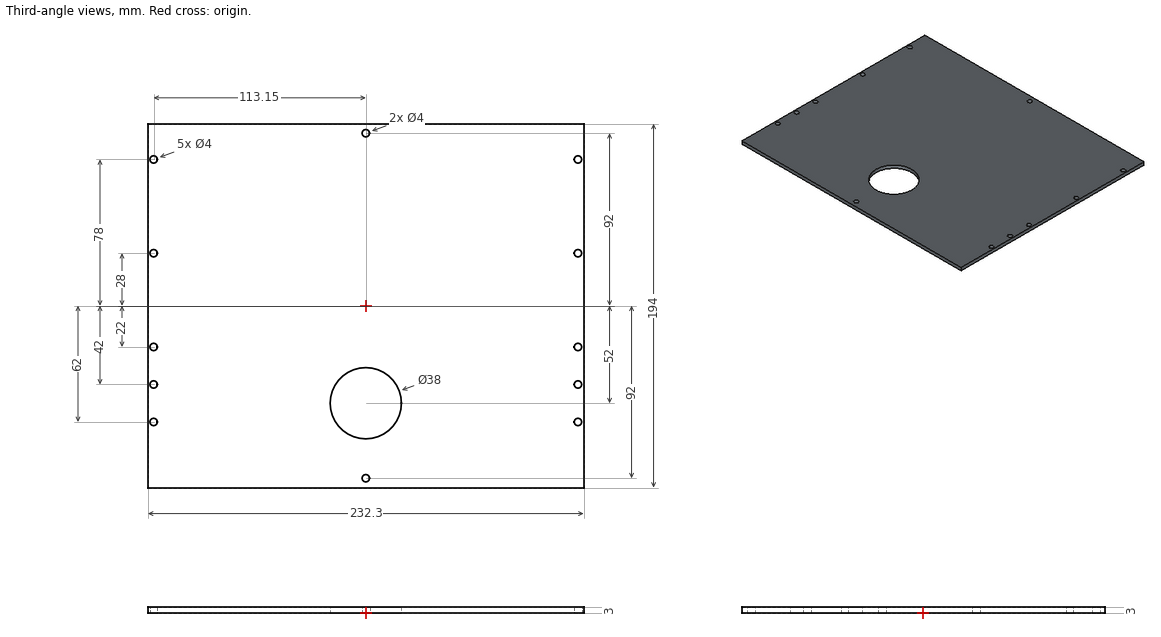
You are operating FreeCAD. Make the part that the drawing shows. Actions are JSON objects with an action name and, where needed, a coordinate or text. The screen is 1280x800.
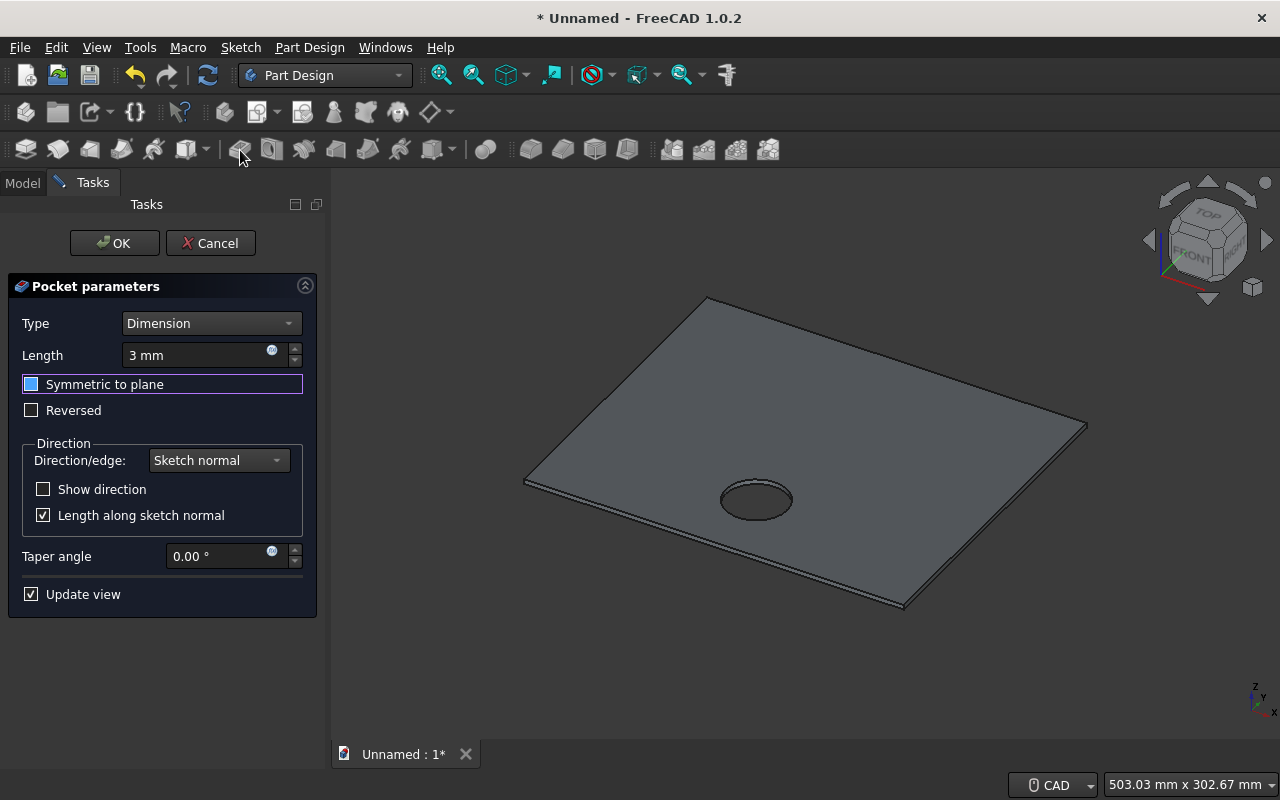
{"action": "left_click", "coordinate": [115, 243]}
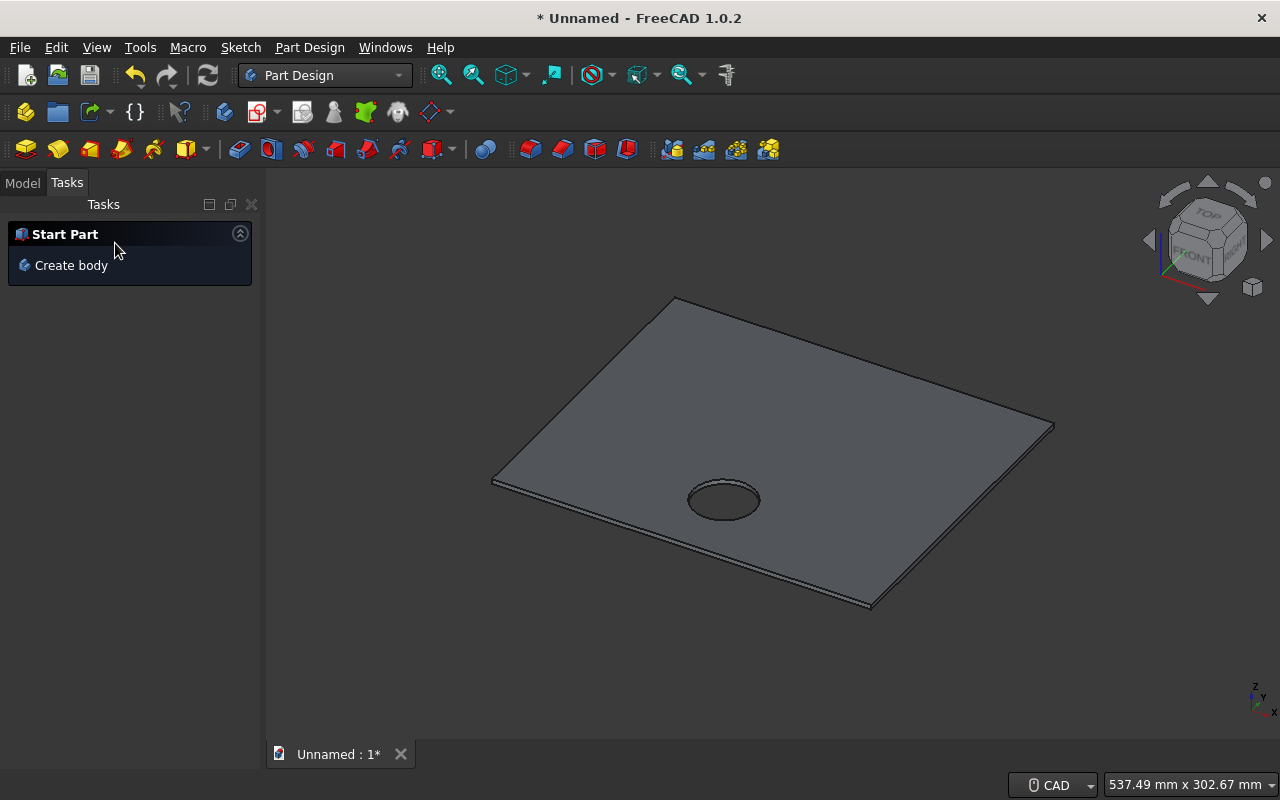
{"action": "left_click", "coordinate": [853, 442]}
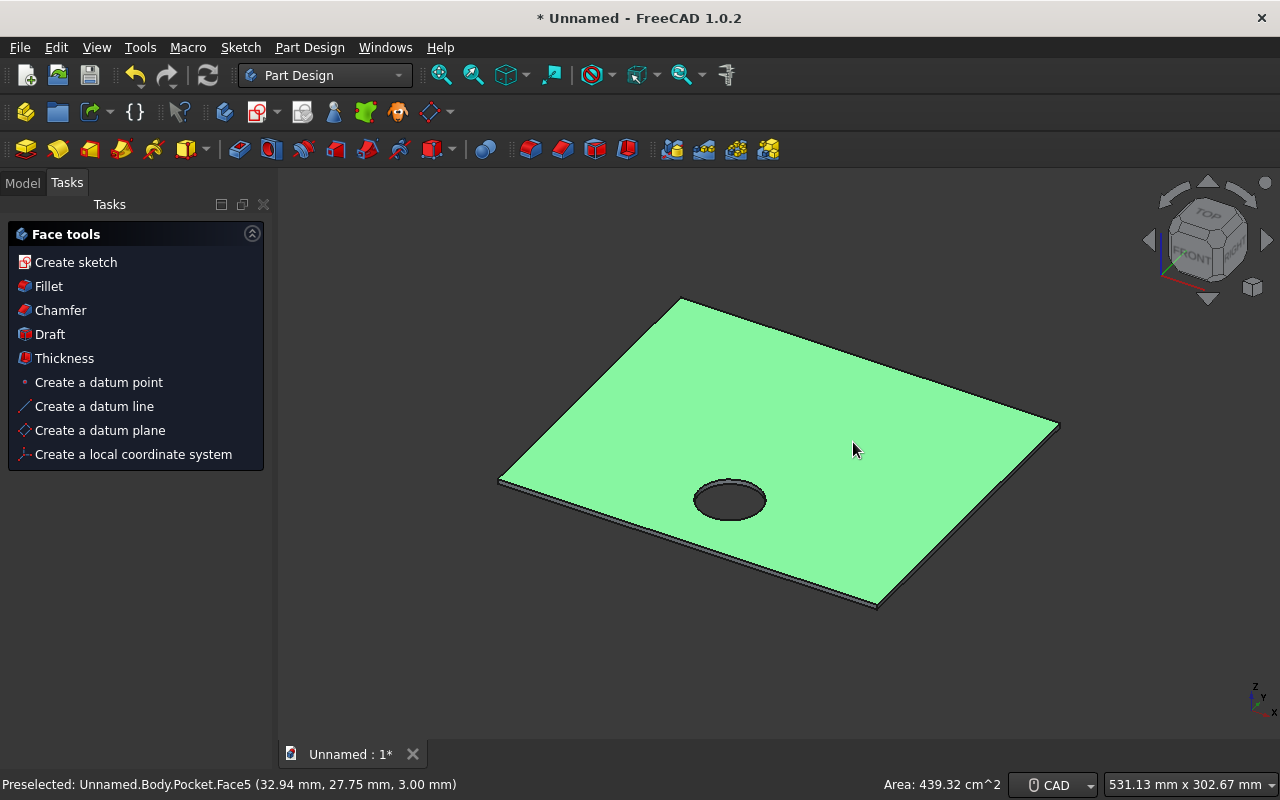
{"action": "left_click", "coordinate": [258, 112]}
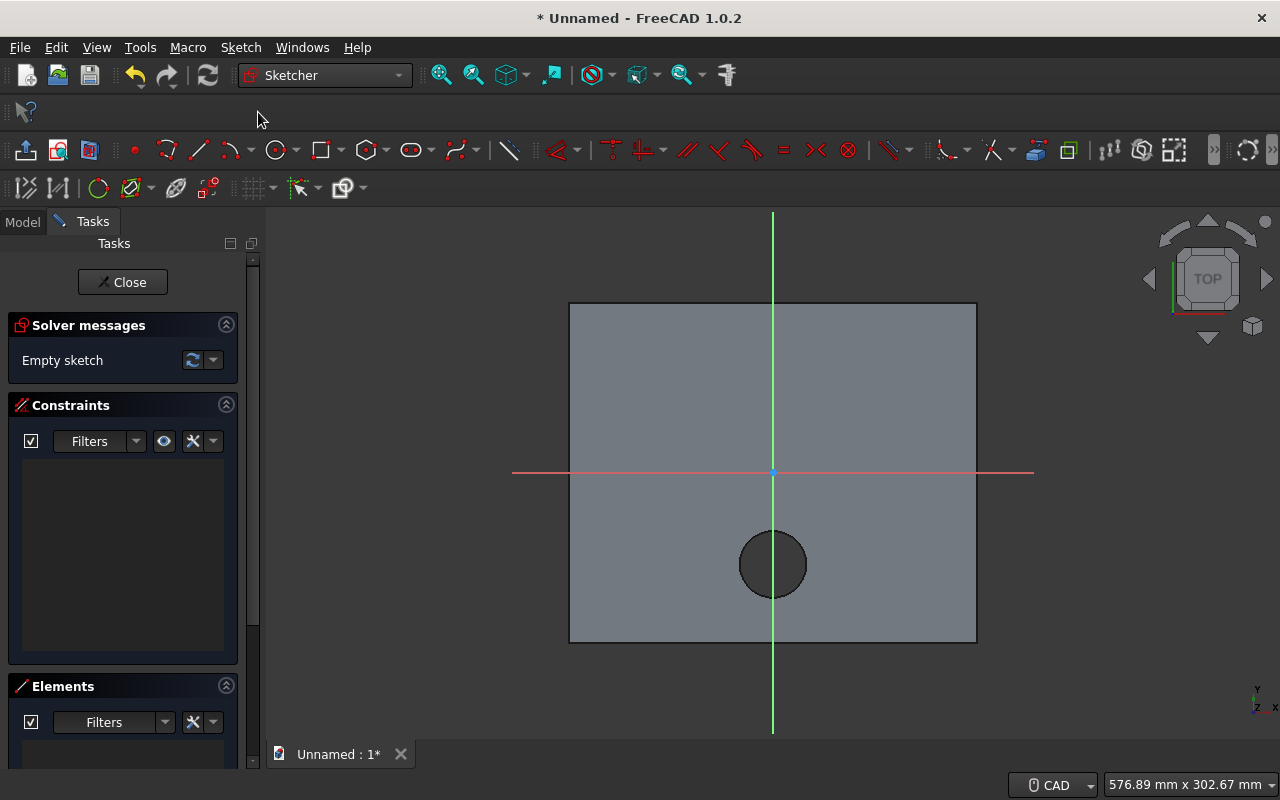
{"action": "key", "text": "g c"}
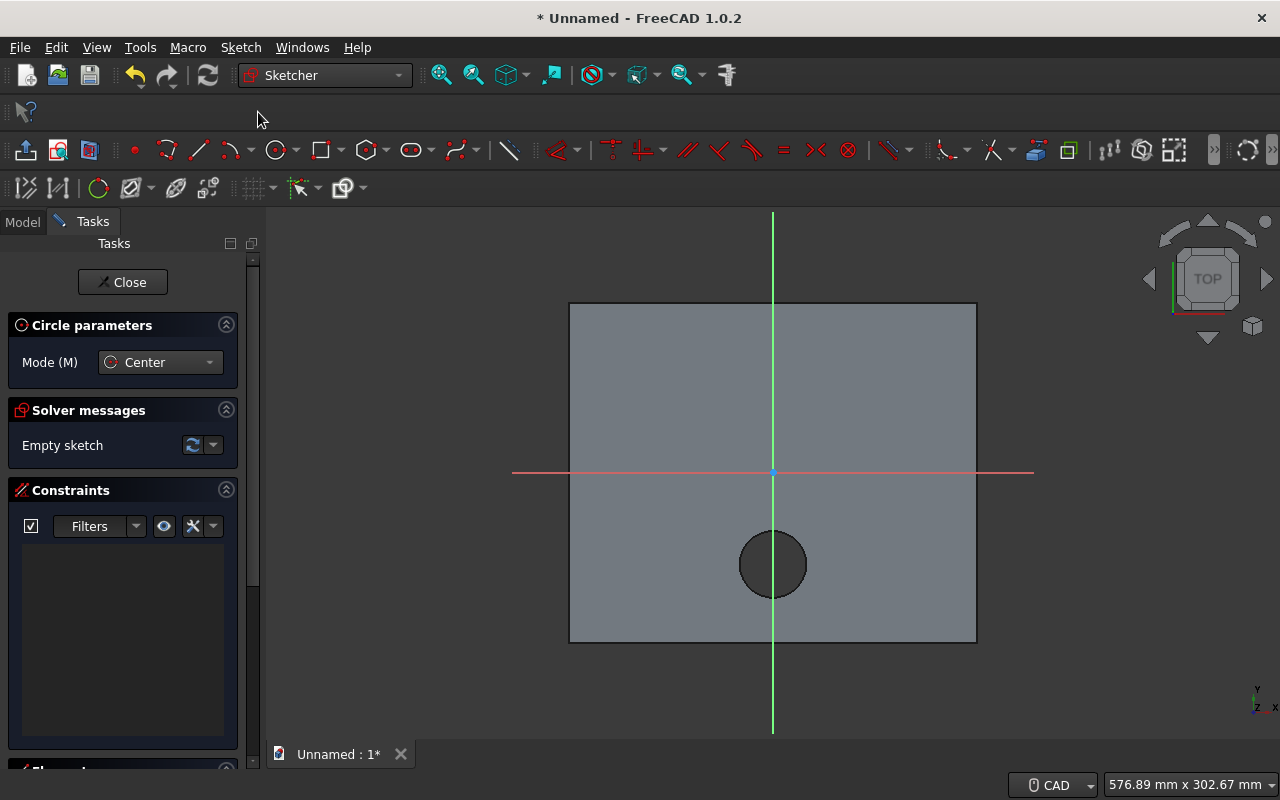
{"action": "scroll", "coordinate": [773, 311], "scroll_direction": "up", "scroll_amount": 10}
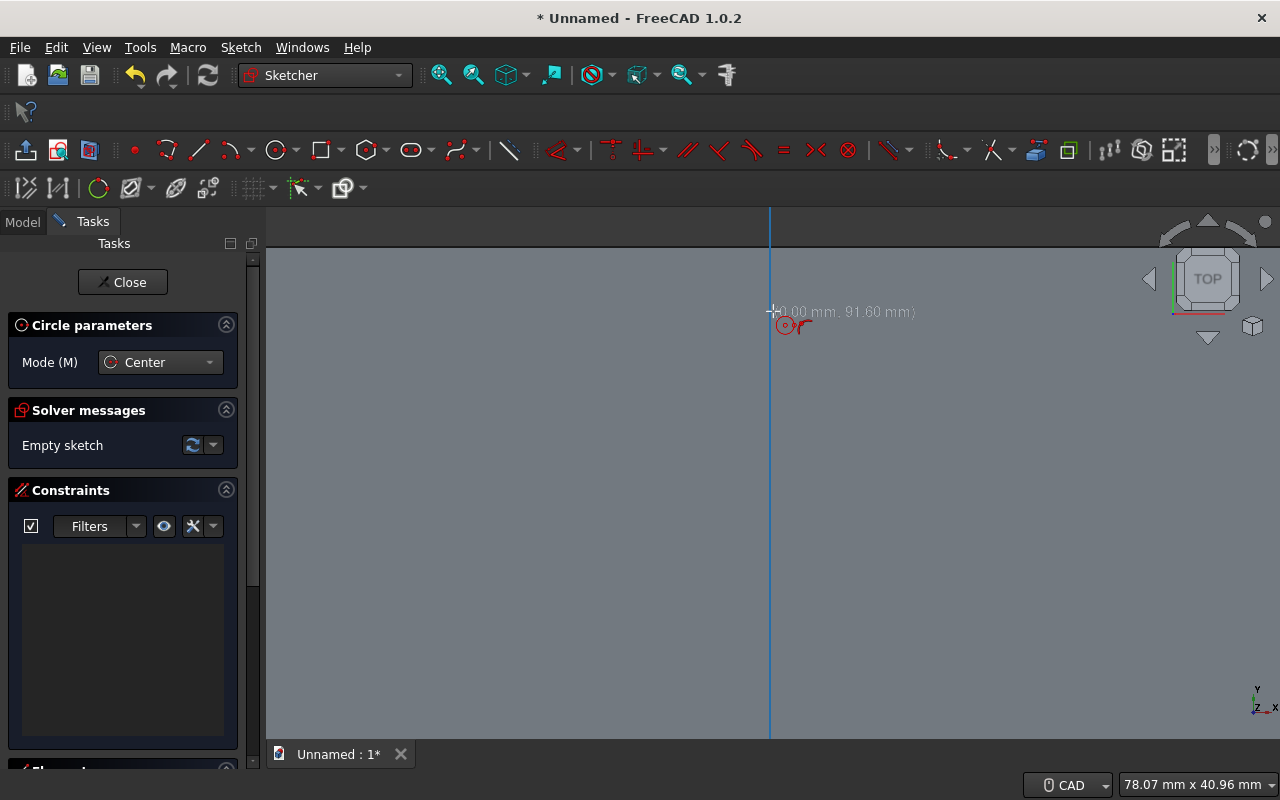
{"action": "scroll", "coordinate": [694, 311], "scroll_direction": "down", "scroll_amount": 10}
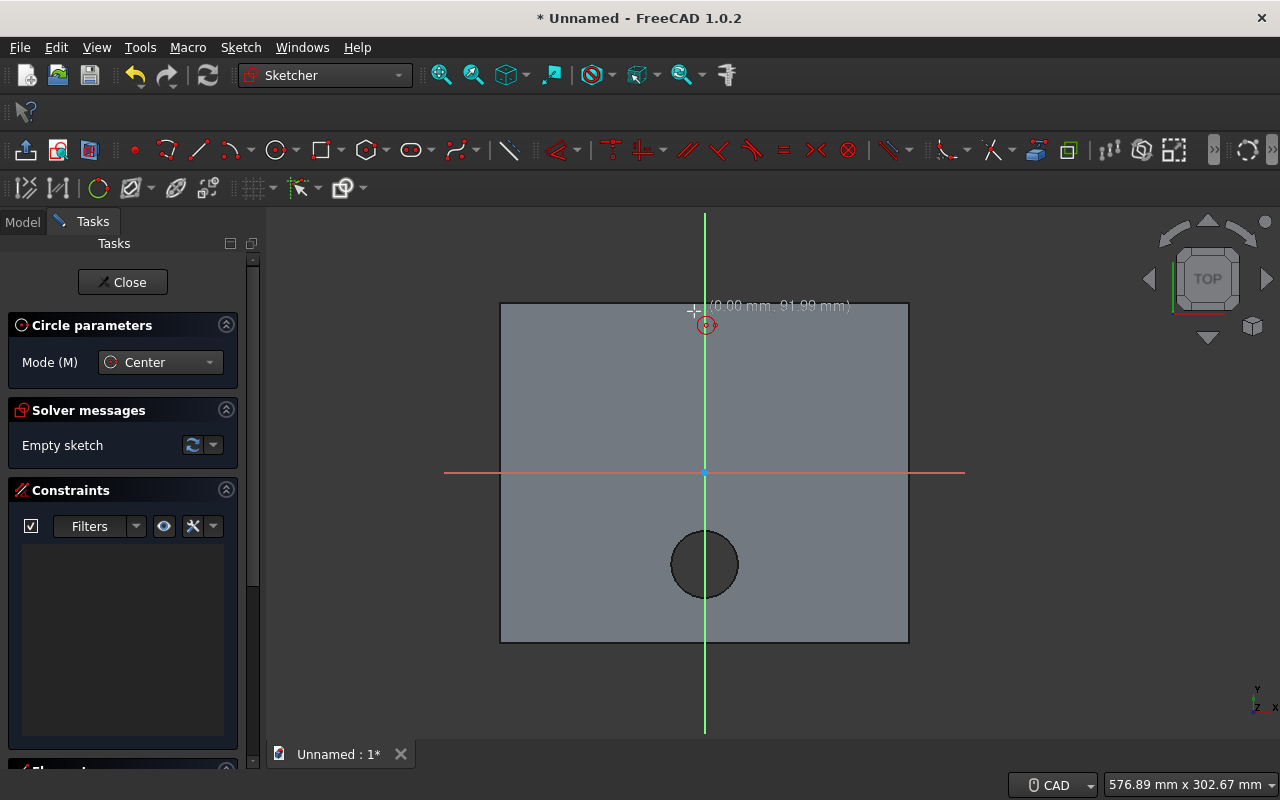
{"action": "left_click", "coordinate": [705, 311]}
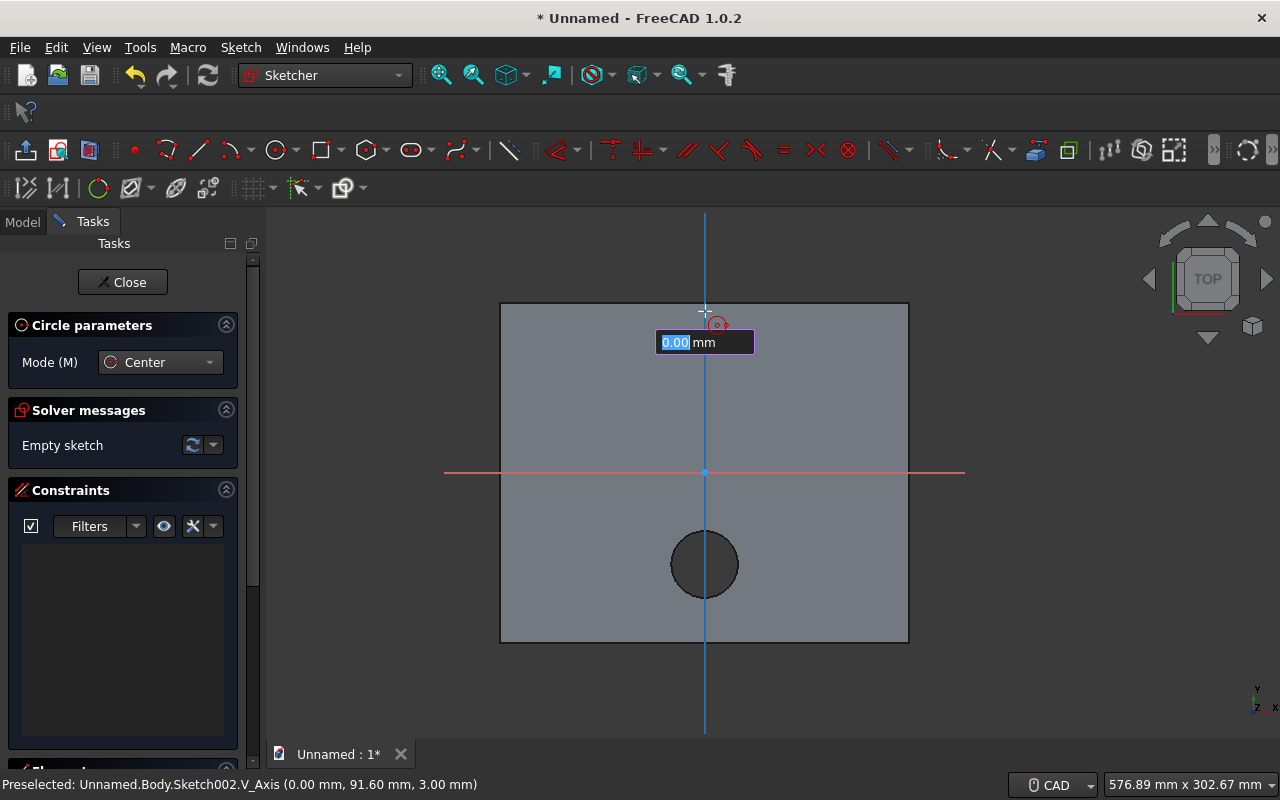
{"action": "scroll", "coordinate": [708, 310], "scroll_direction": "up", "scroll_amount": 8}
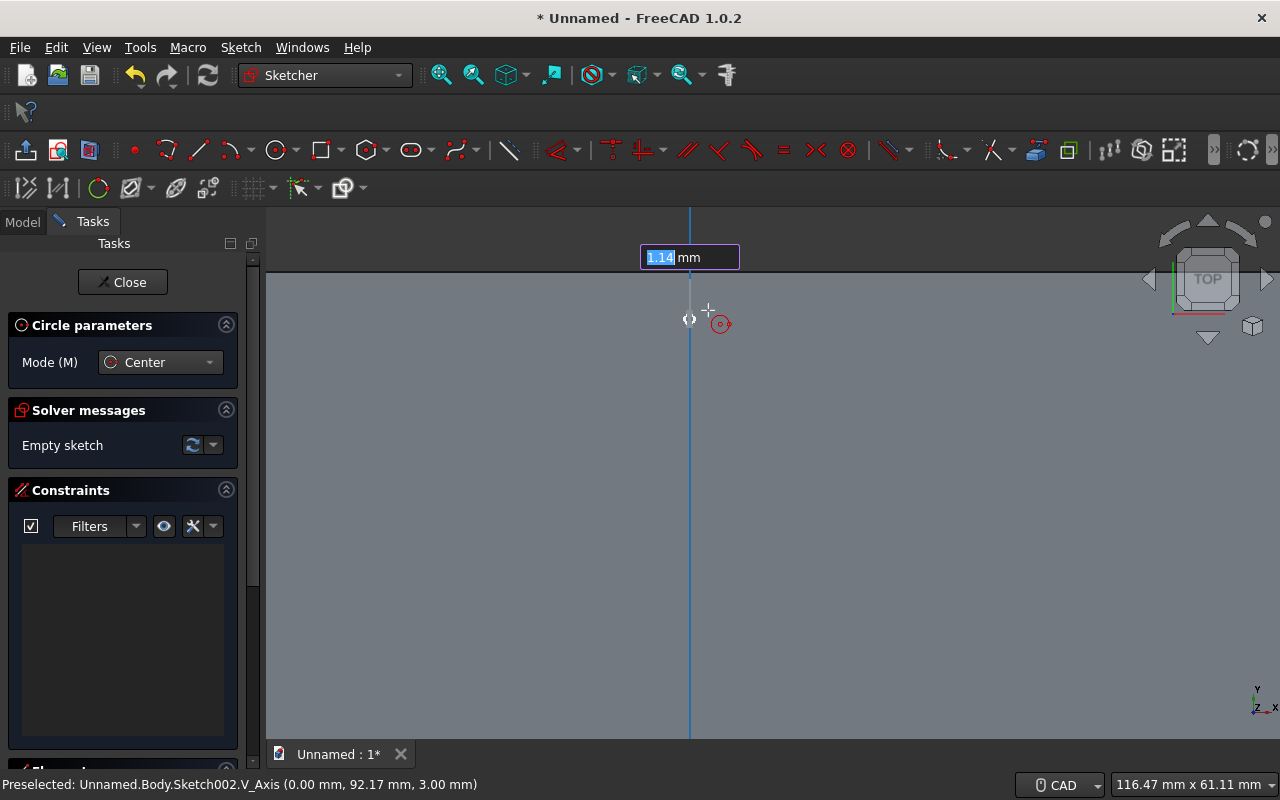
{"action": "left_click", "coordinate": [706, 310]}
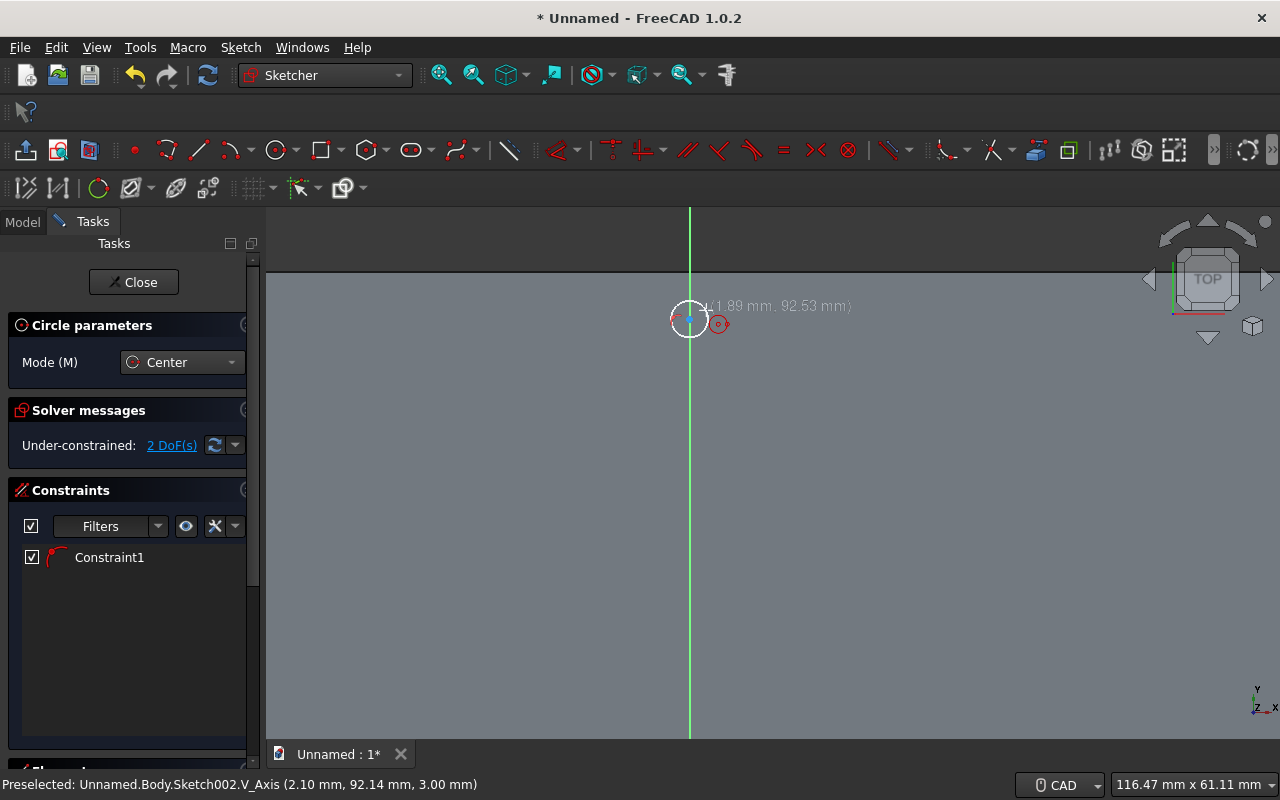
{"action": "scroll", "coordinate": [708, 310], "scroll_direction": "down", "scroll_amount": 8}